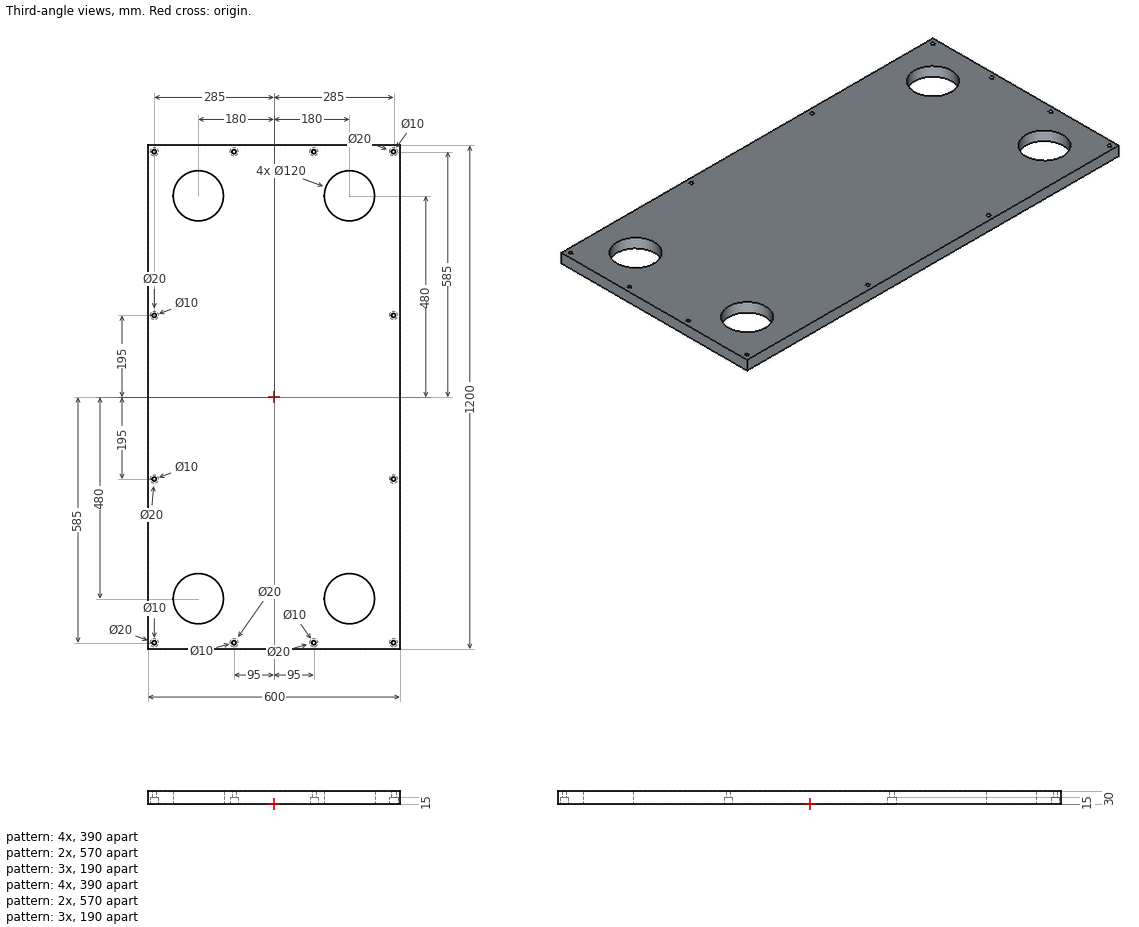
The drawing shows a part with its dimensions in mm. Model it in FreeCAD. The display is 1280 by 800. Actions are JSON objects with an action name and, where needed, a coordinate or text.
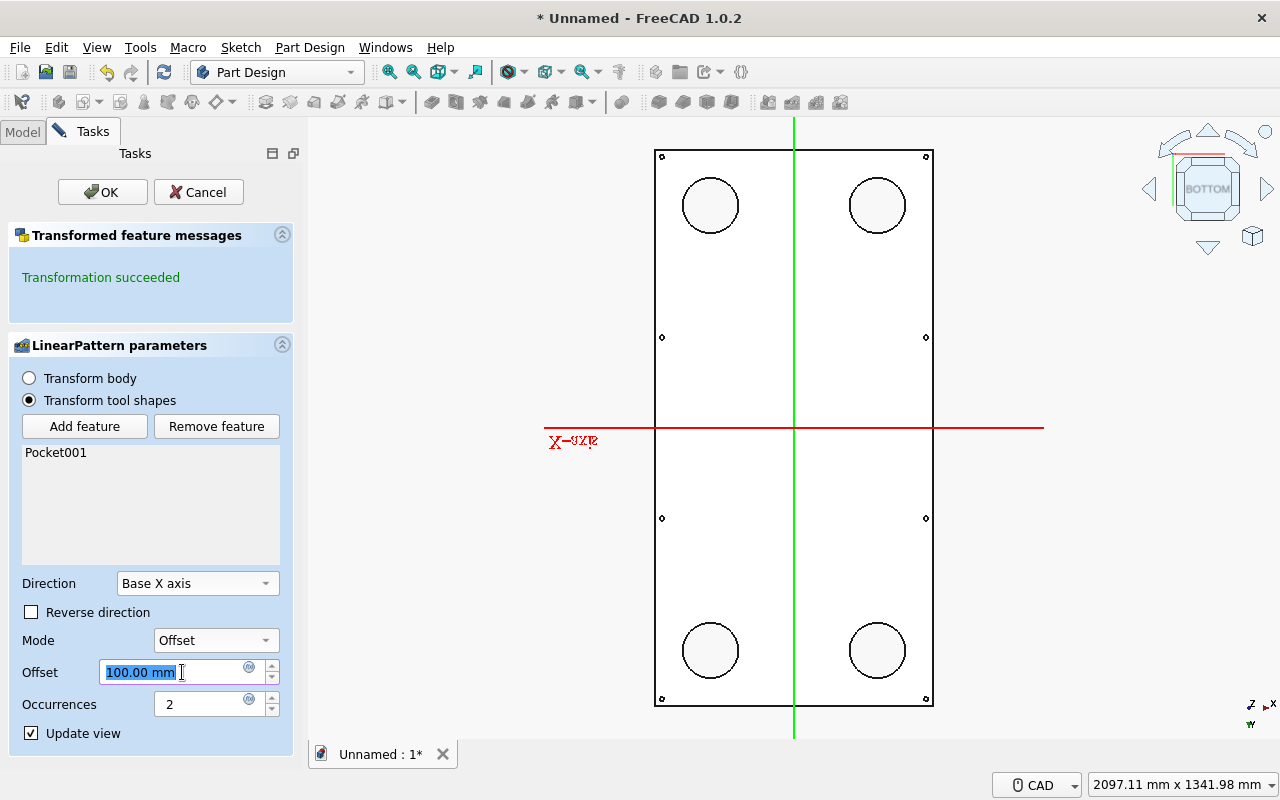
{"action": "type", "text": "190"}
{"action": "key", "text": "Tab"}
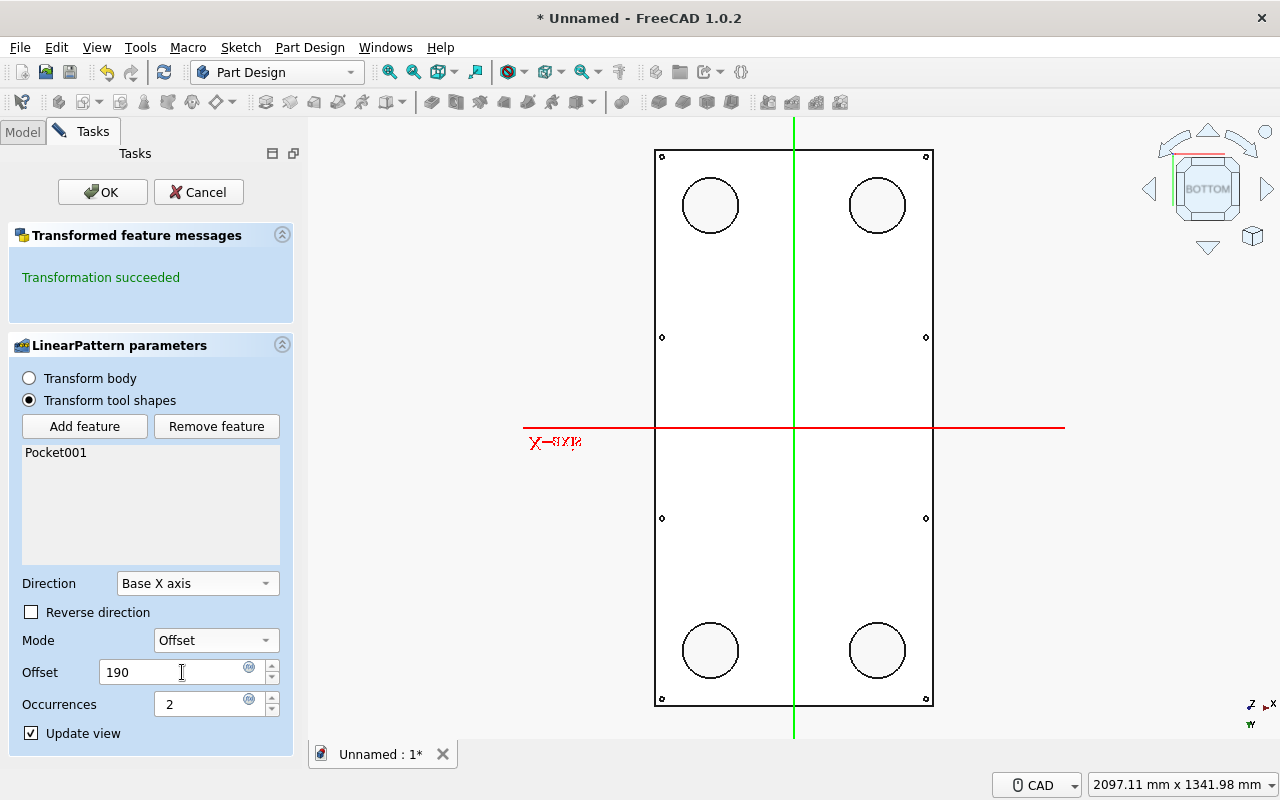
{"action": "triple_click", "coordinate": [209, 704]}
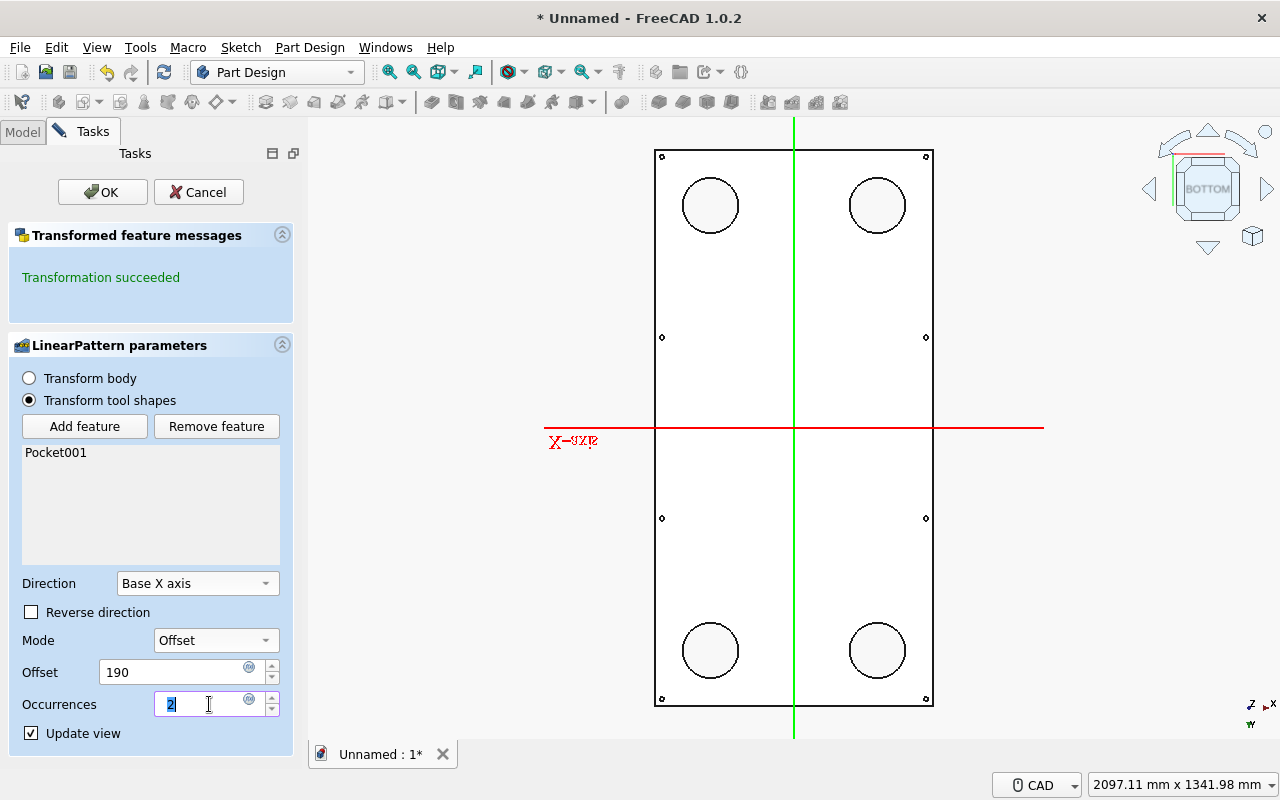
{"action": "type", "text": "3"}
{"action": "key", "text": "Tab"}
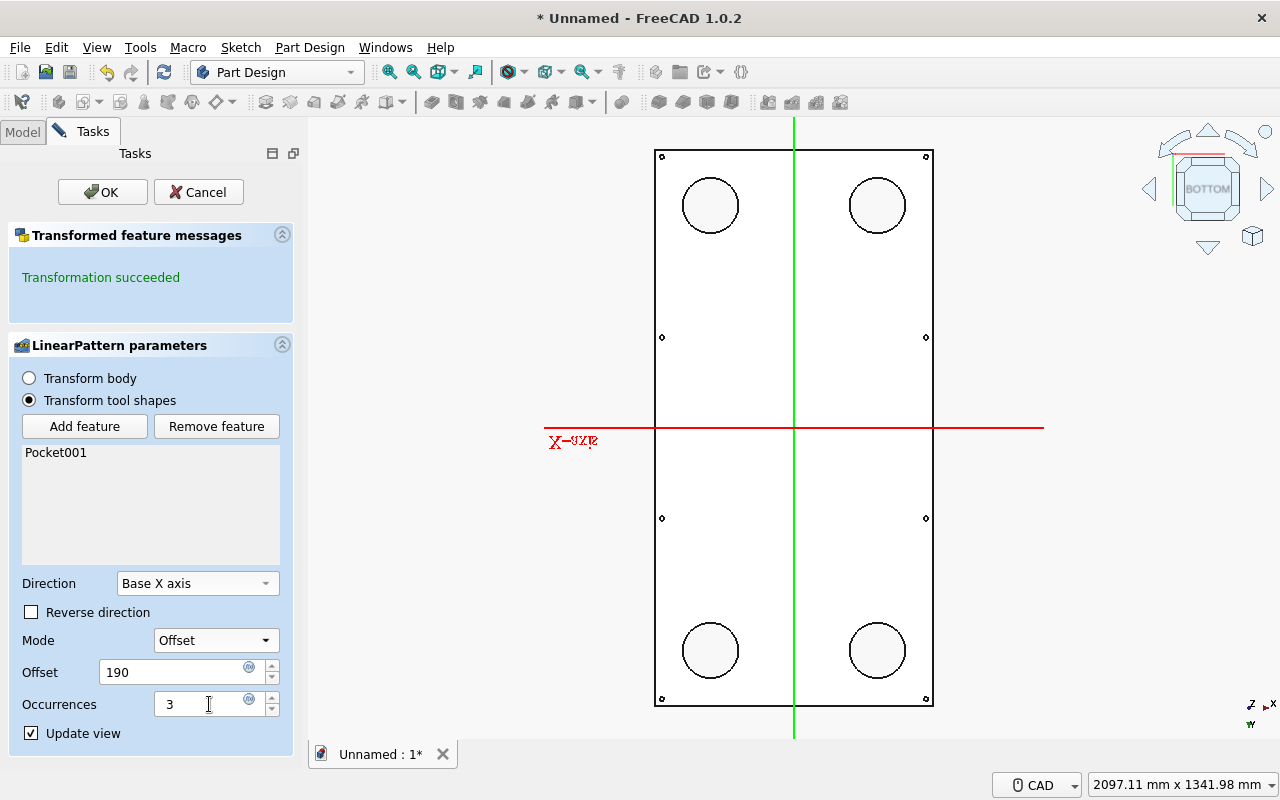
{"action": "left_click", "coordinate": [30, 612]}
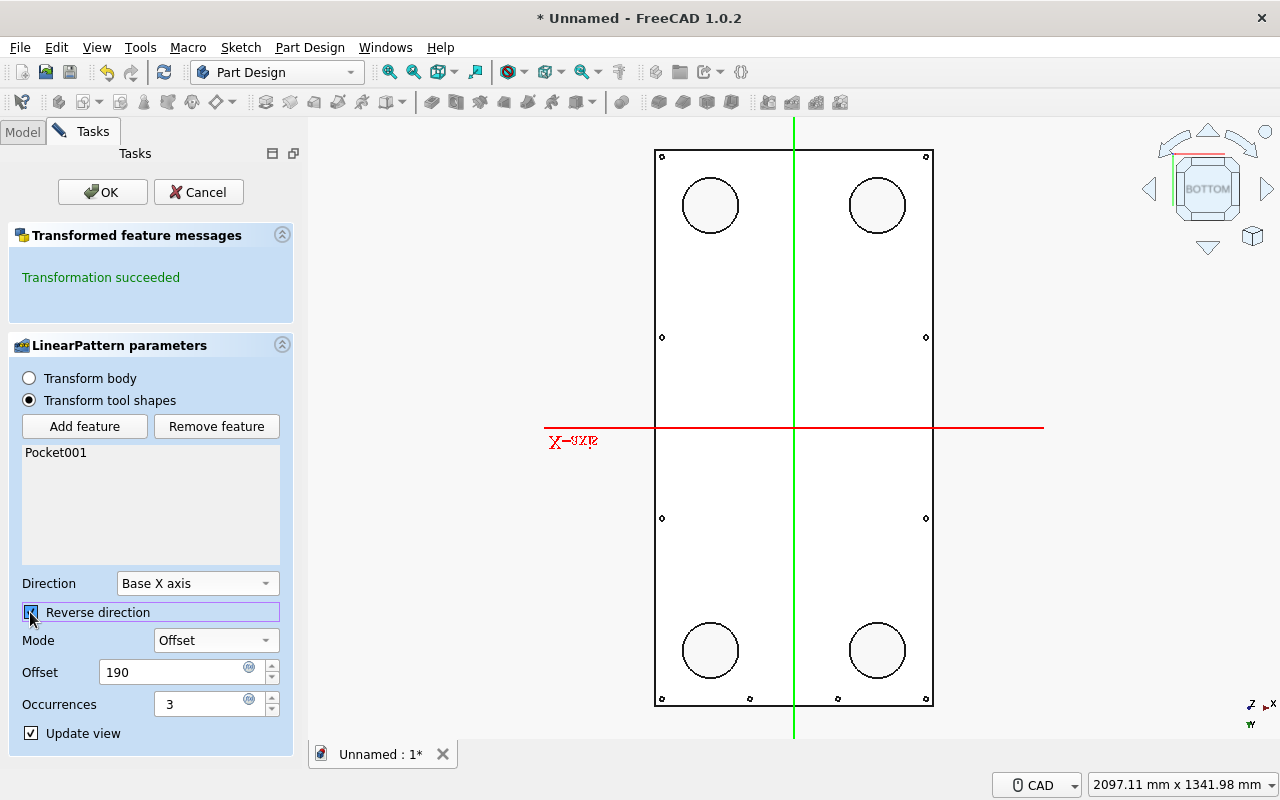
{"action": "left_click", "coordinate": [103, 192]}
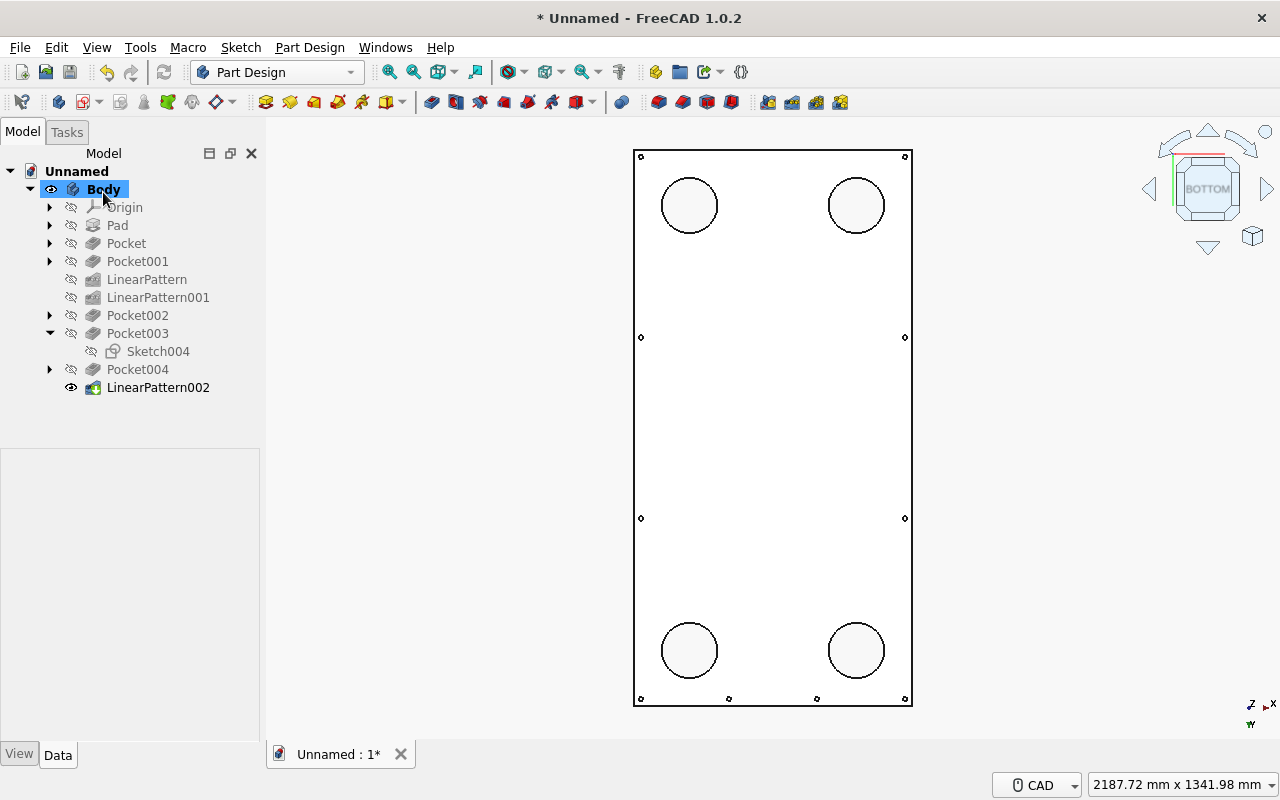
{"action": "left_click", "coordinate": [773, 427]}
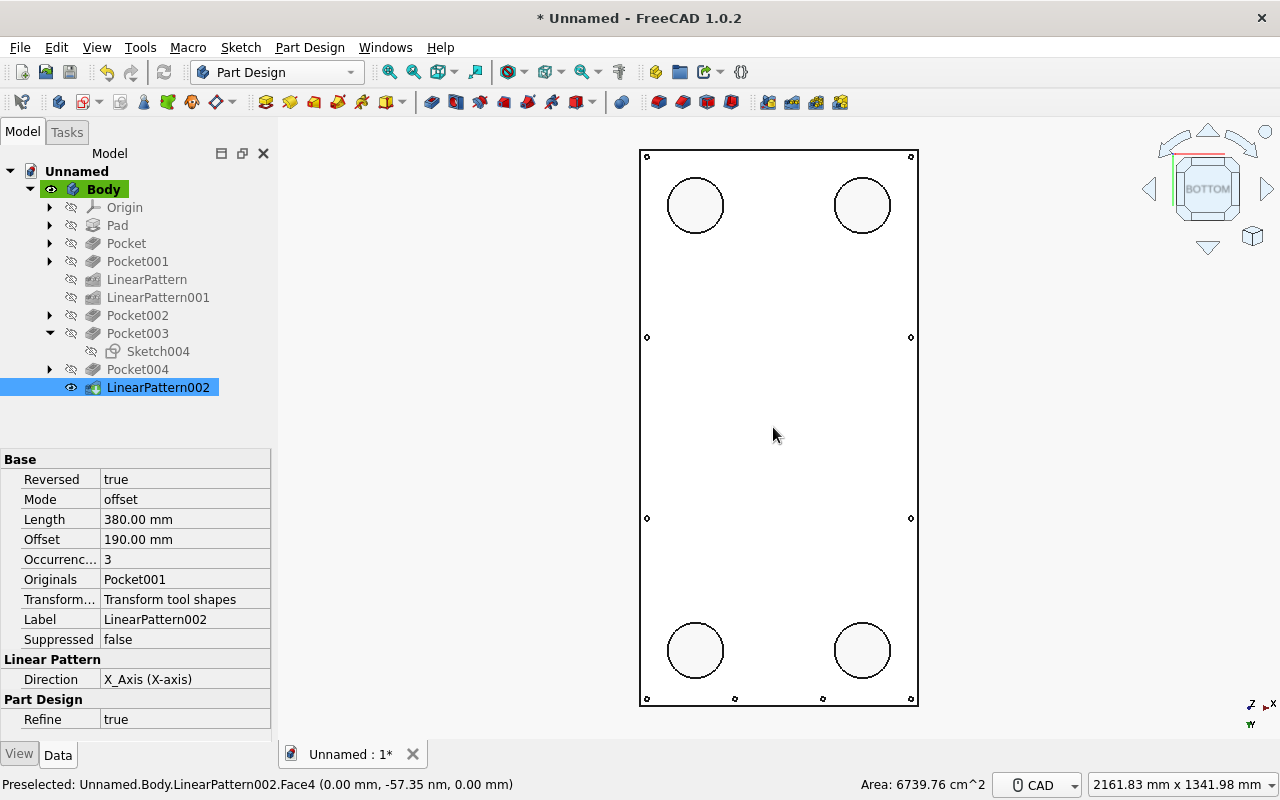
{"action": "left_click", "coordinate": [84, 102]}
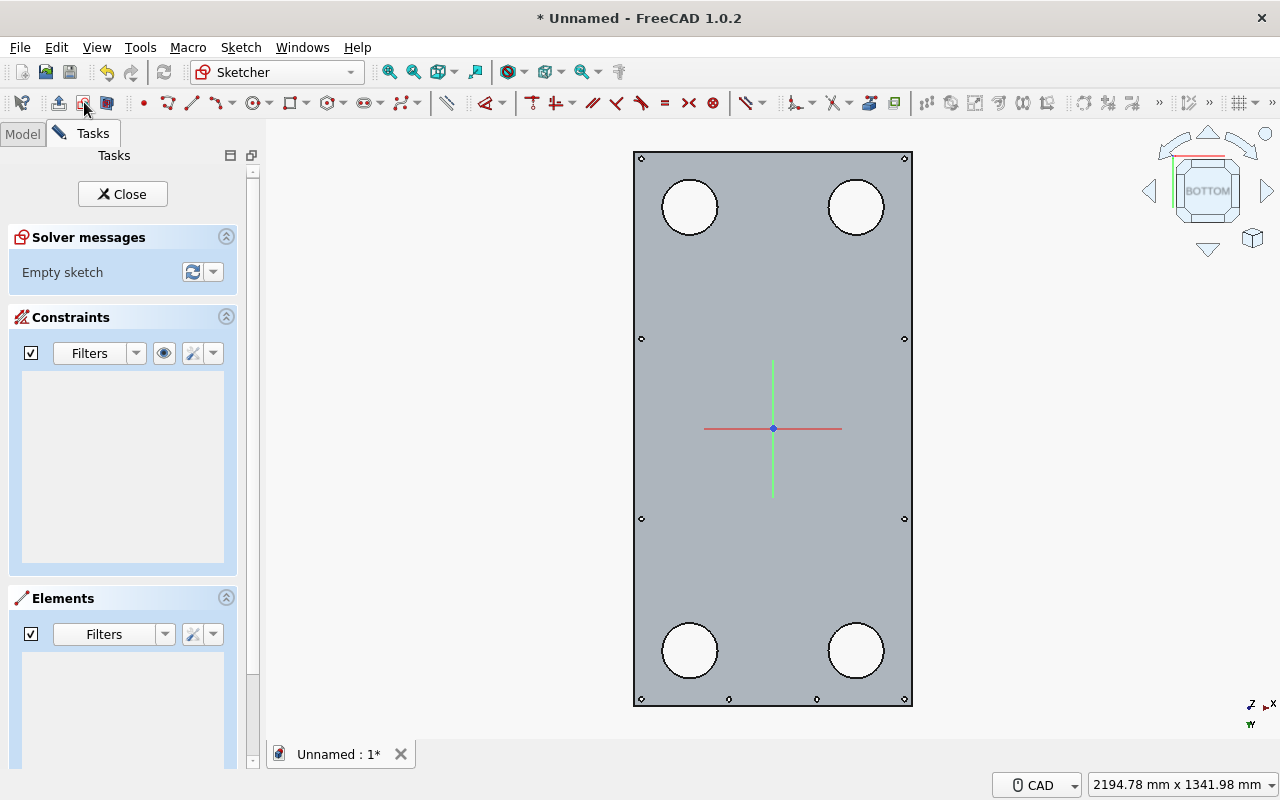
{"action": "scroll", "coordinate": [823, 147], "scroll_direction": "up", "scroll_amount": 15}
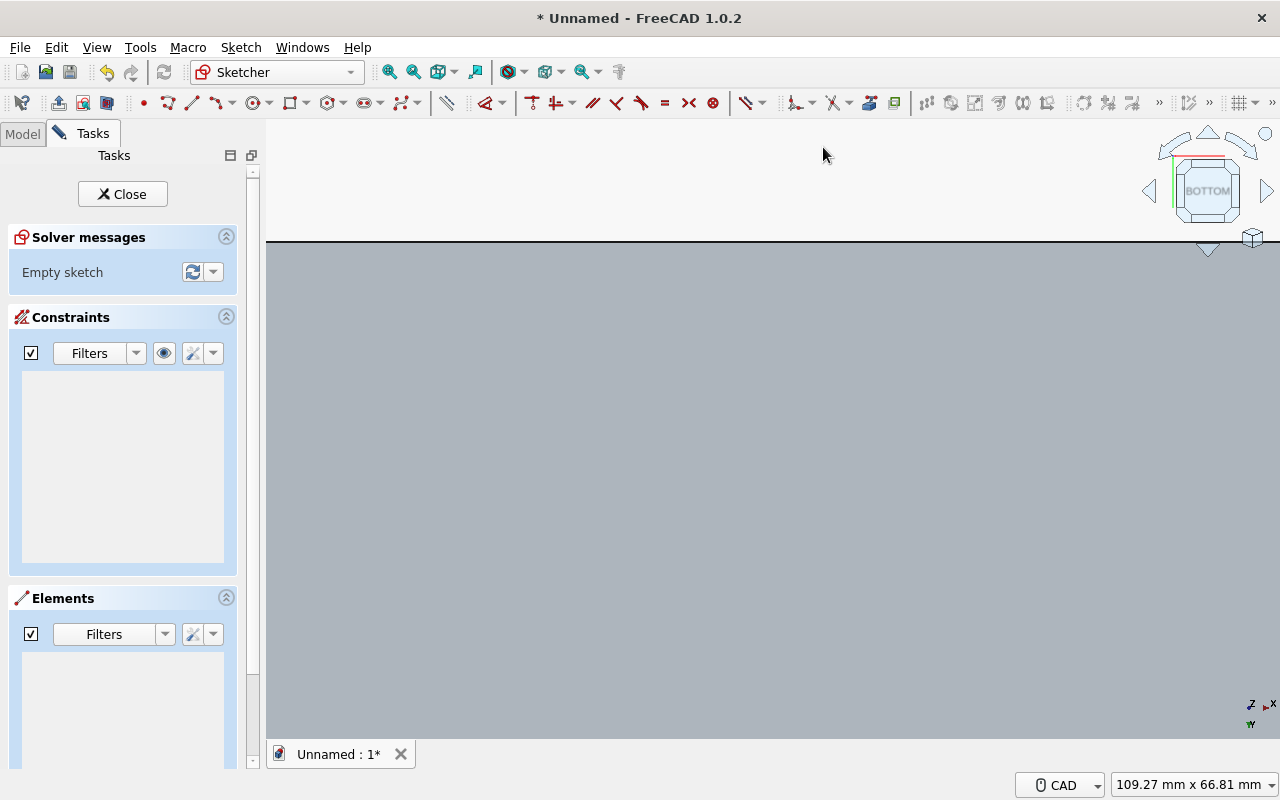
{"action": "scroll", "coordinate": [685, 366], "scroll_direction": "up", "scroll_amount": 7}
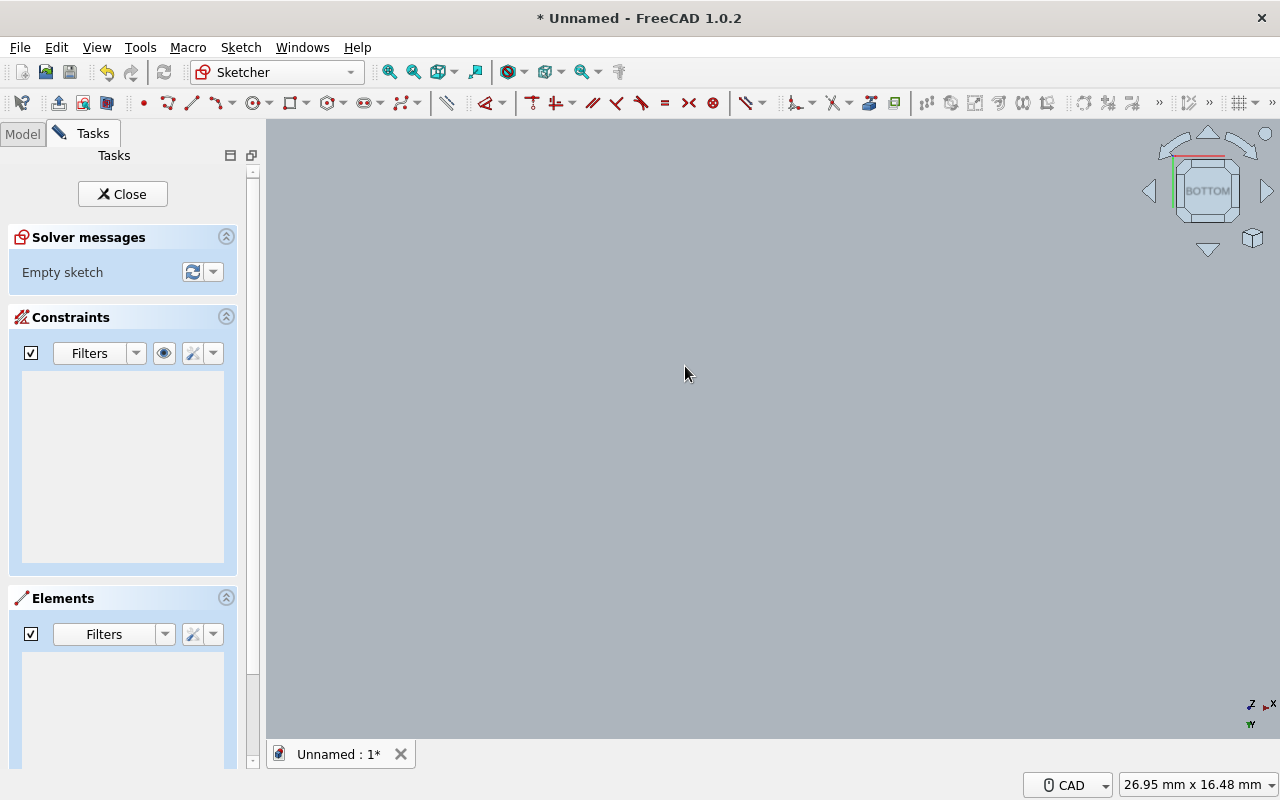
{"action": "left_click", "coordinate": [254, 104]}